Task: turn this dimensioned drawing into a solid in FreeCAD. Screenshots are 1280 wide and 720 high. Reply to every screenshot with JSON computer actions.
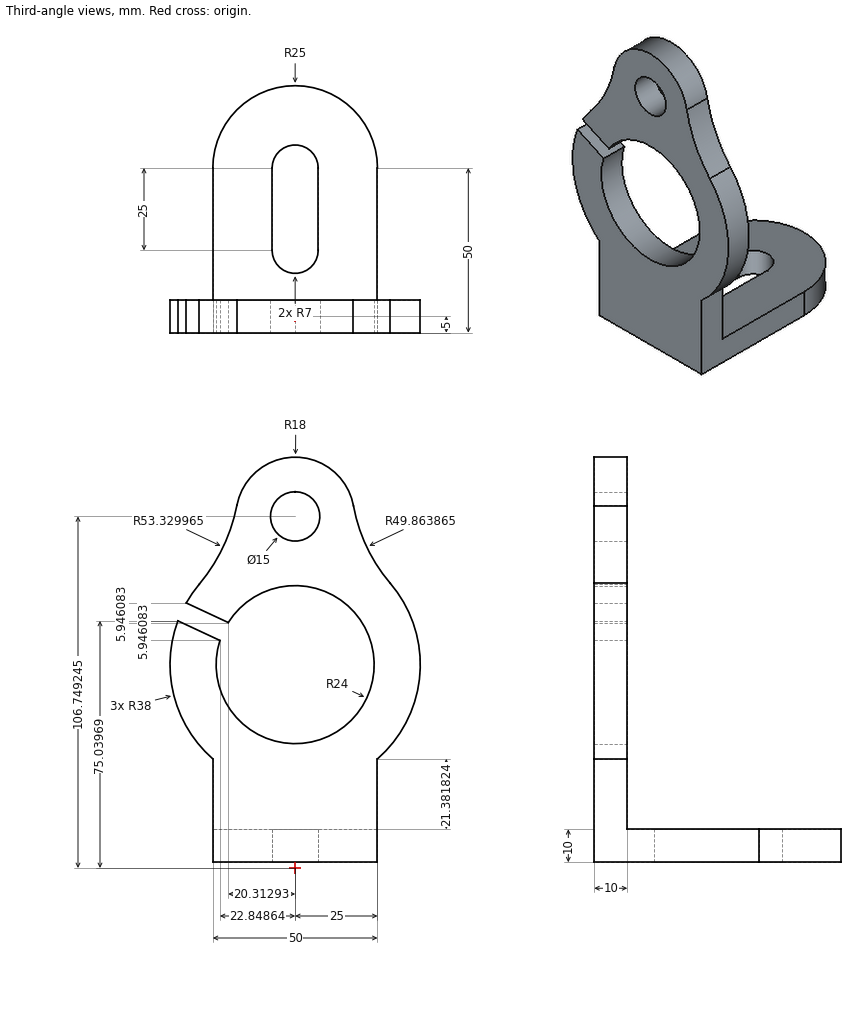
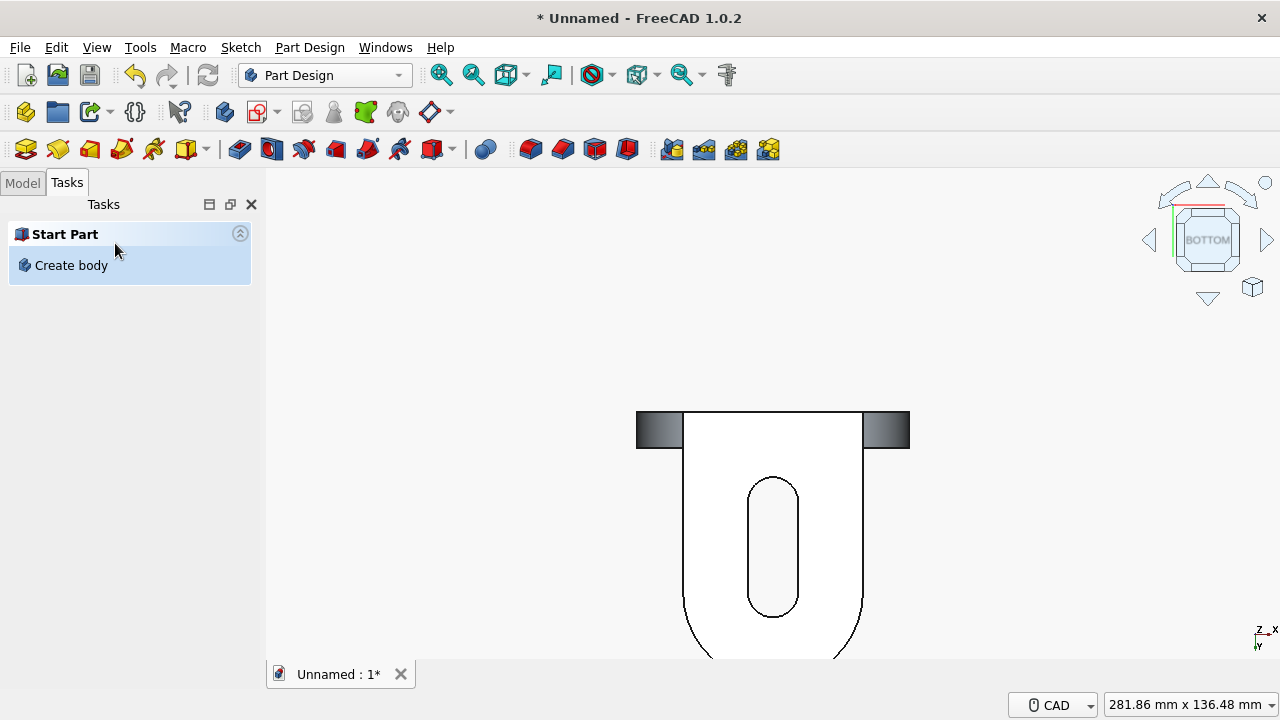
{"action": "key", "text": "0"}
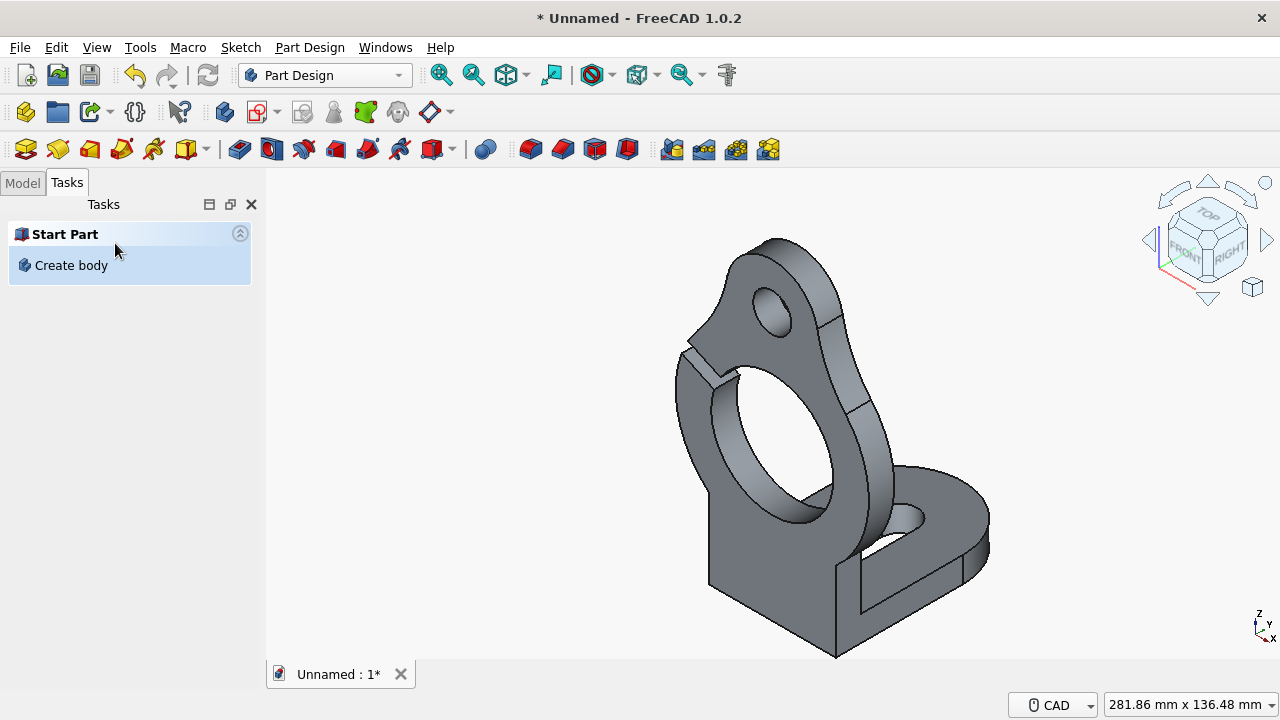
{"action": "key", "text": "v f"}